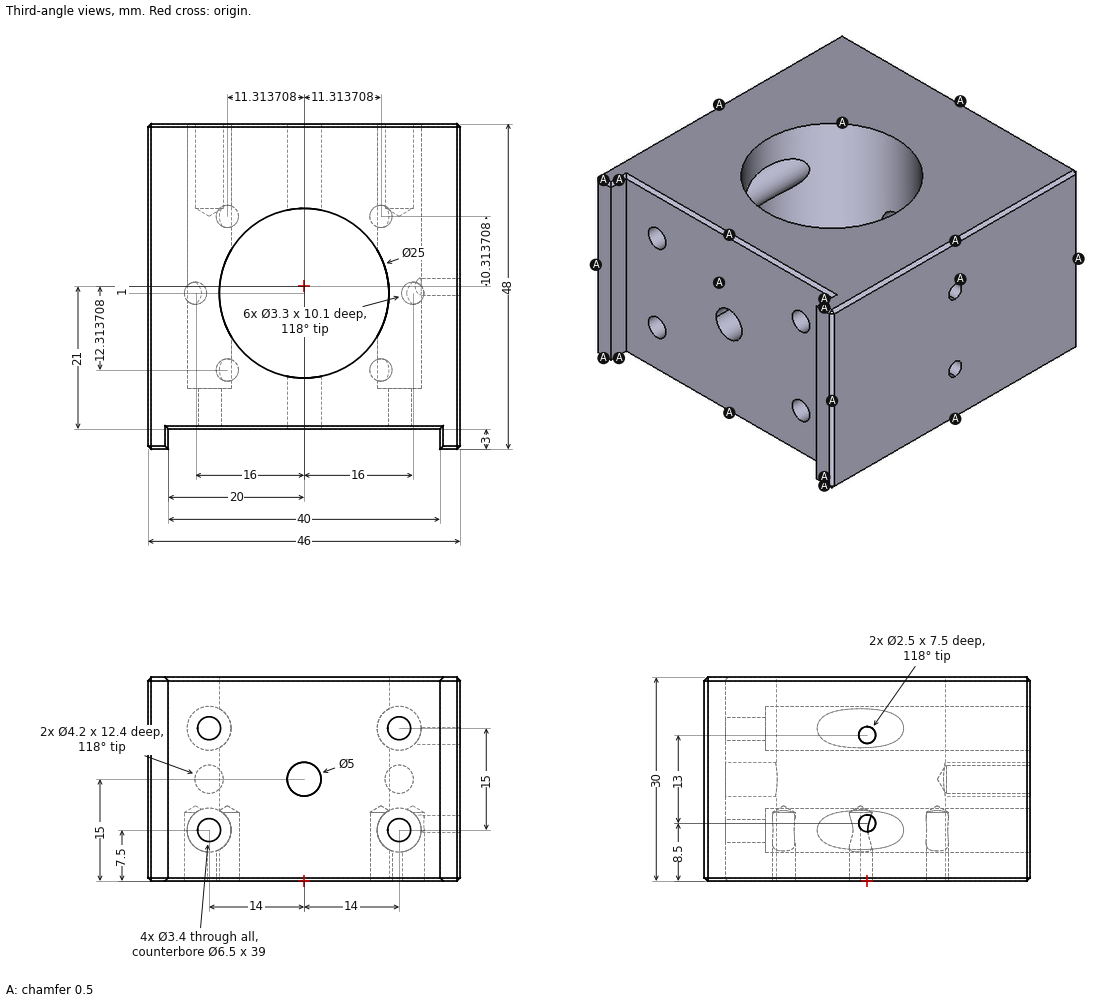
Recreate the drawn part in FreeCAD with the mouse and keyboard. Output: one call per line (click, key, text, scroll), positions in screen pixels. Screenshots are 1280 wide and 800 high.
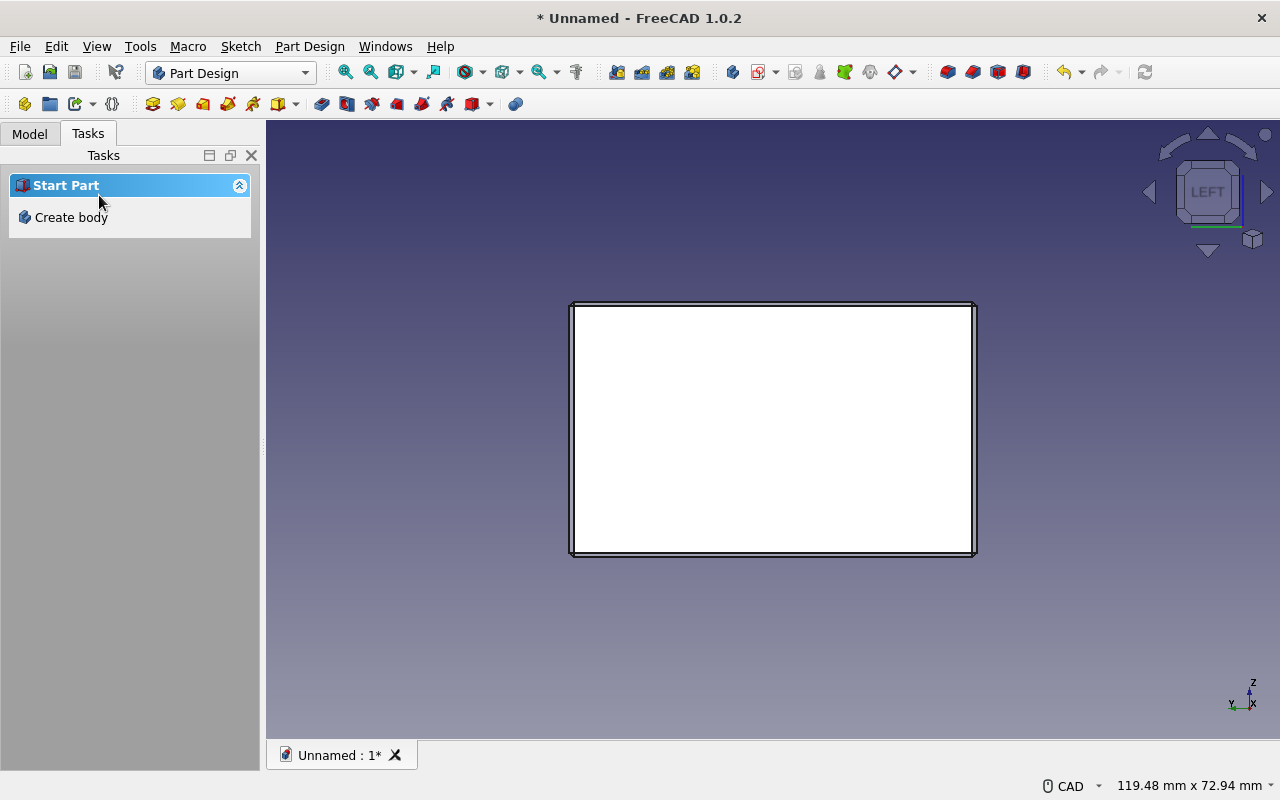
click(346, 72)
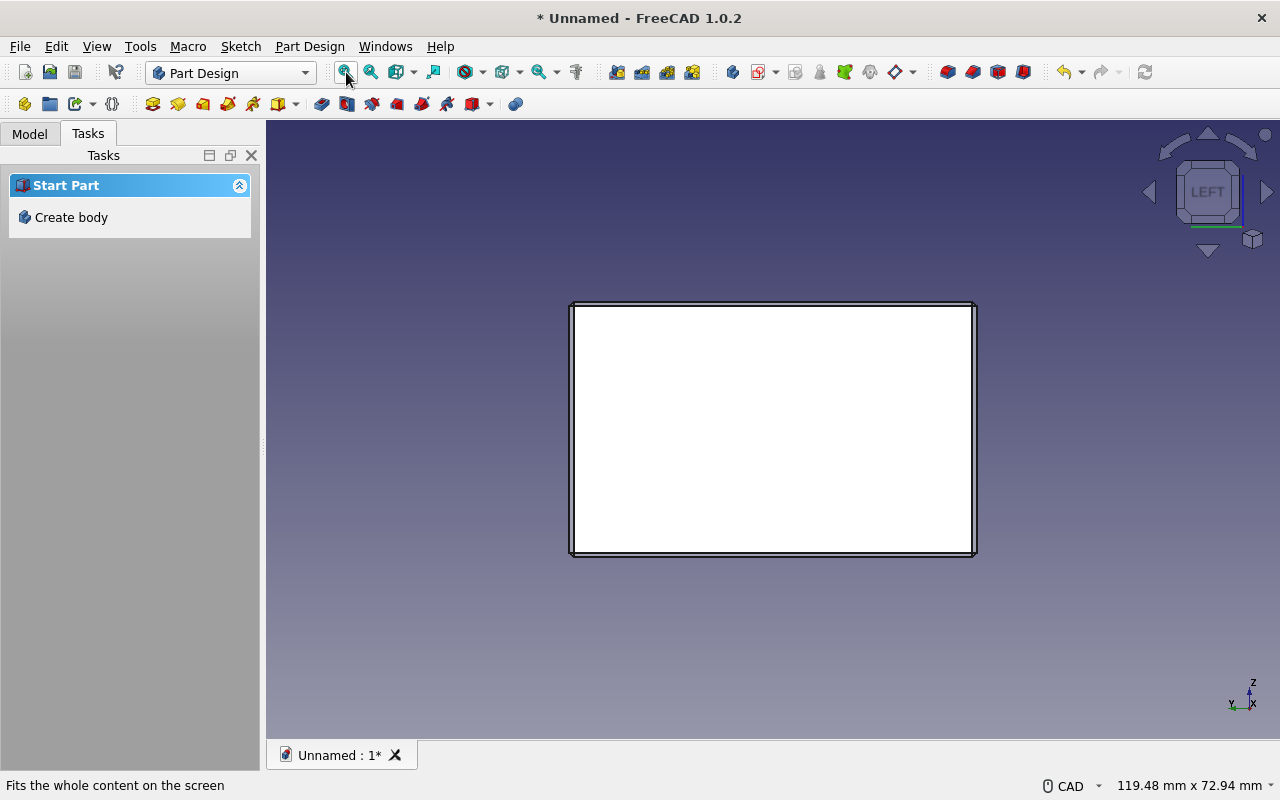
key(4)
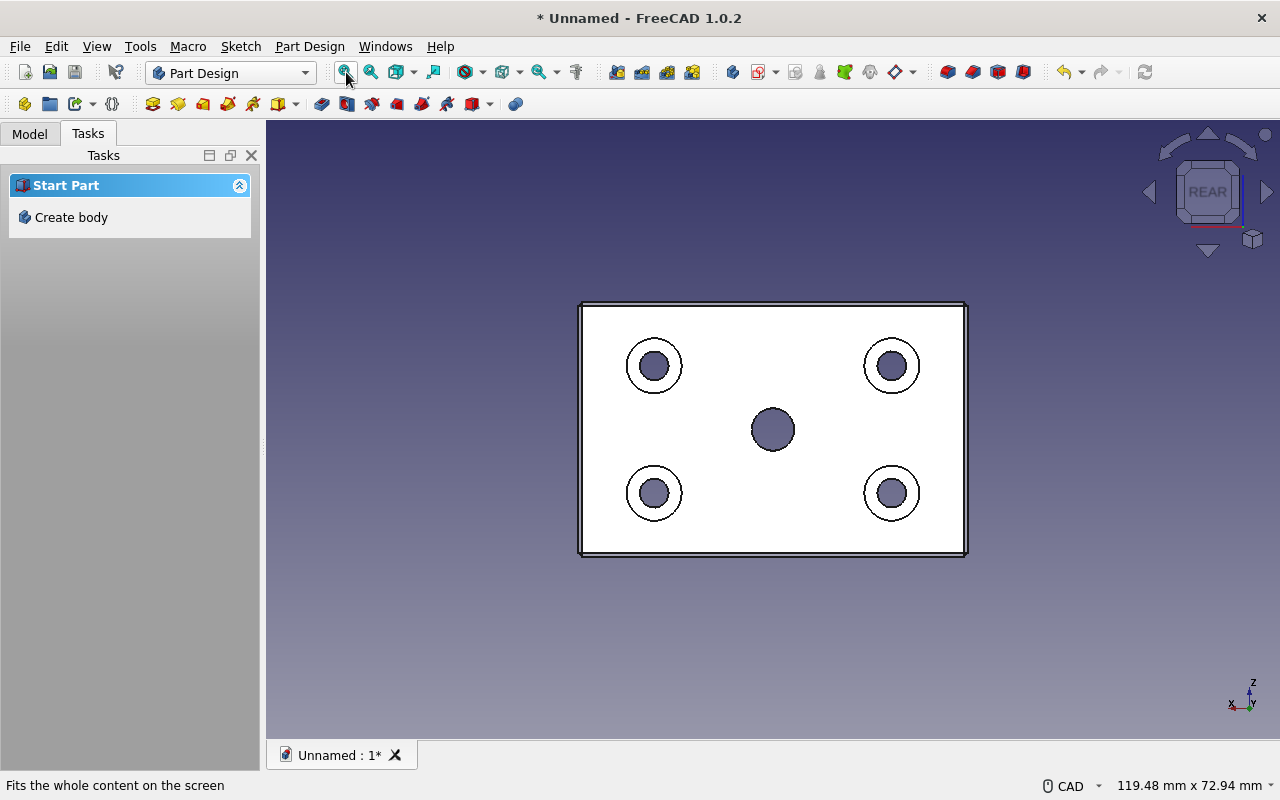
click(346, 72)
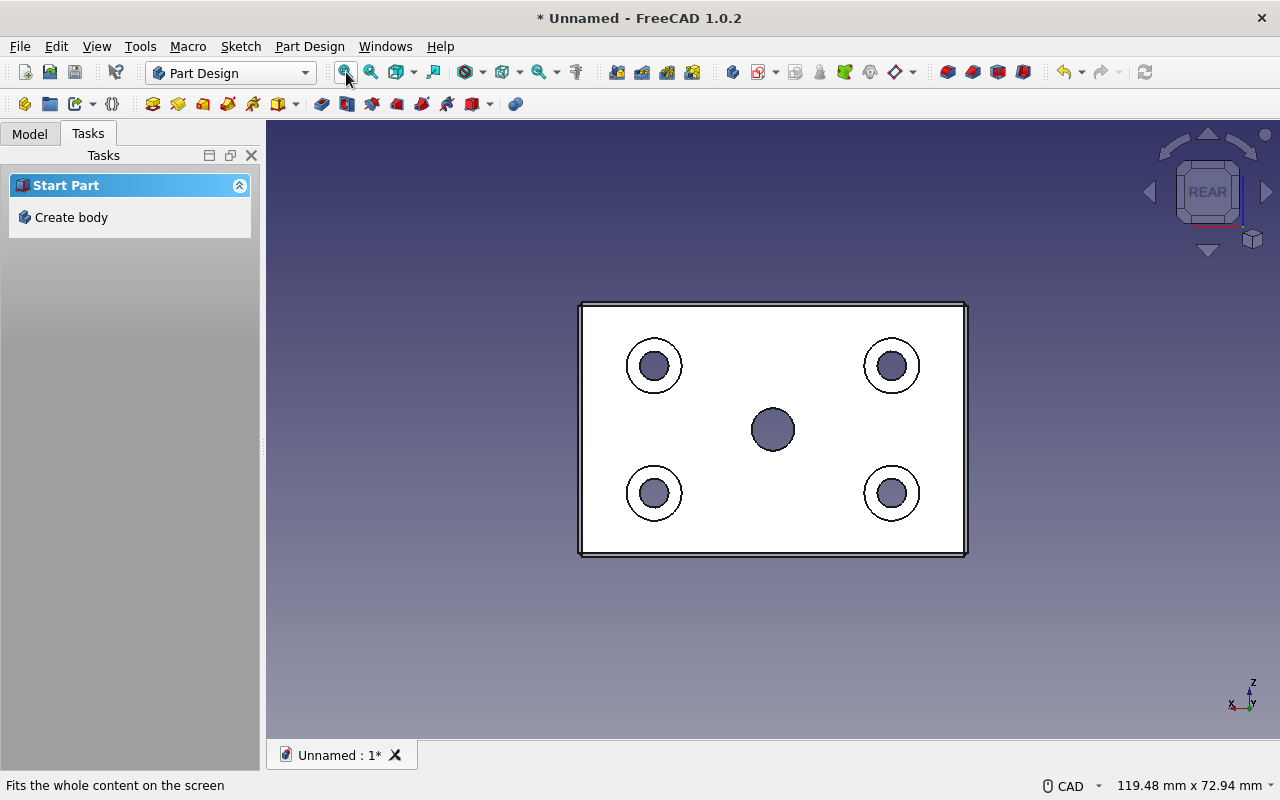
click(773, 358)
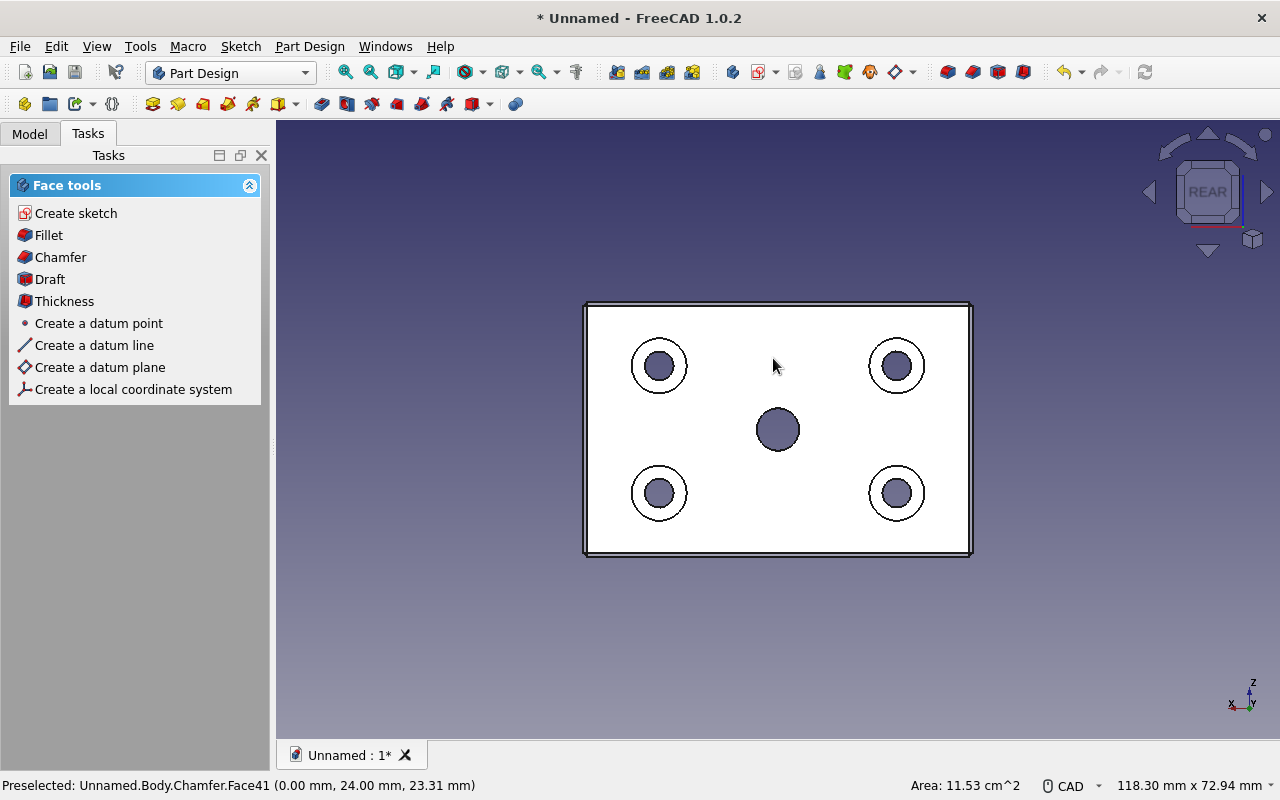
click(758, 72)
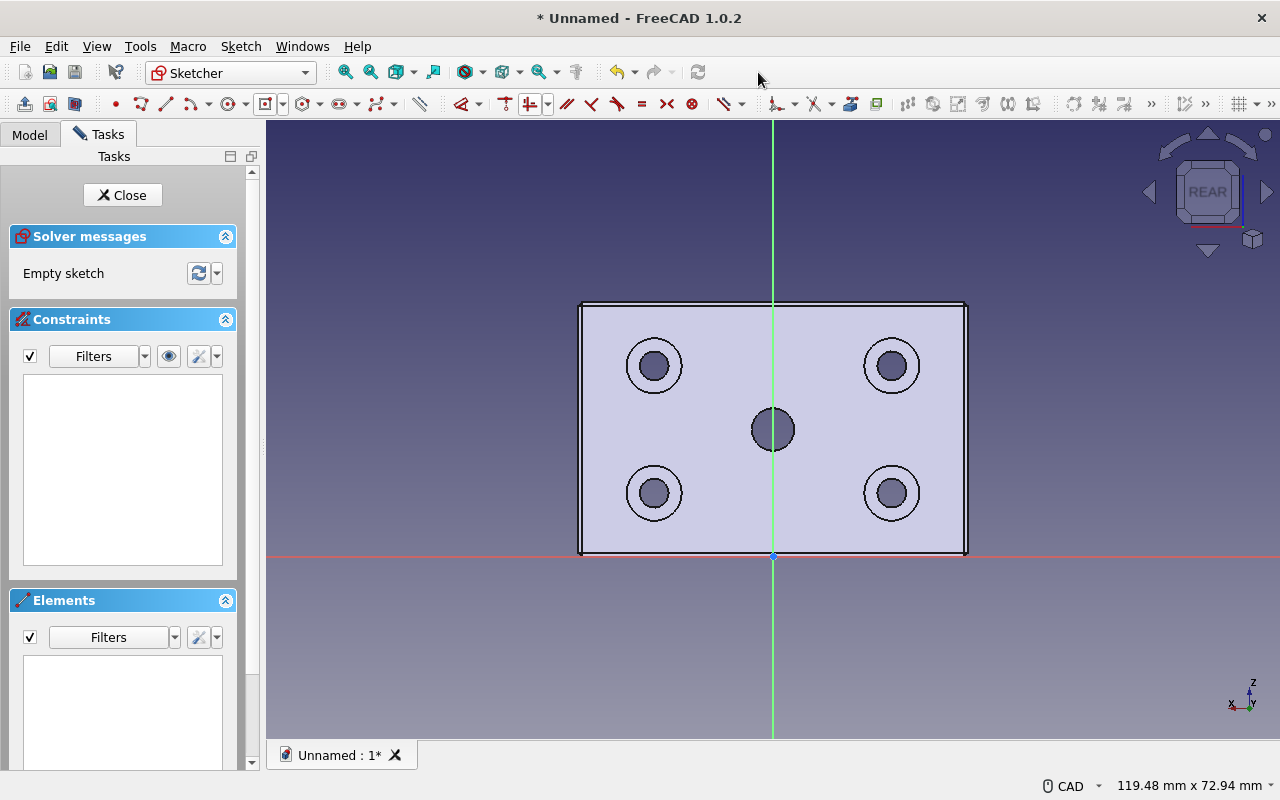
scroll(829, 529, up, 4)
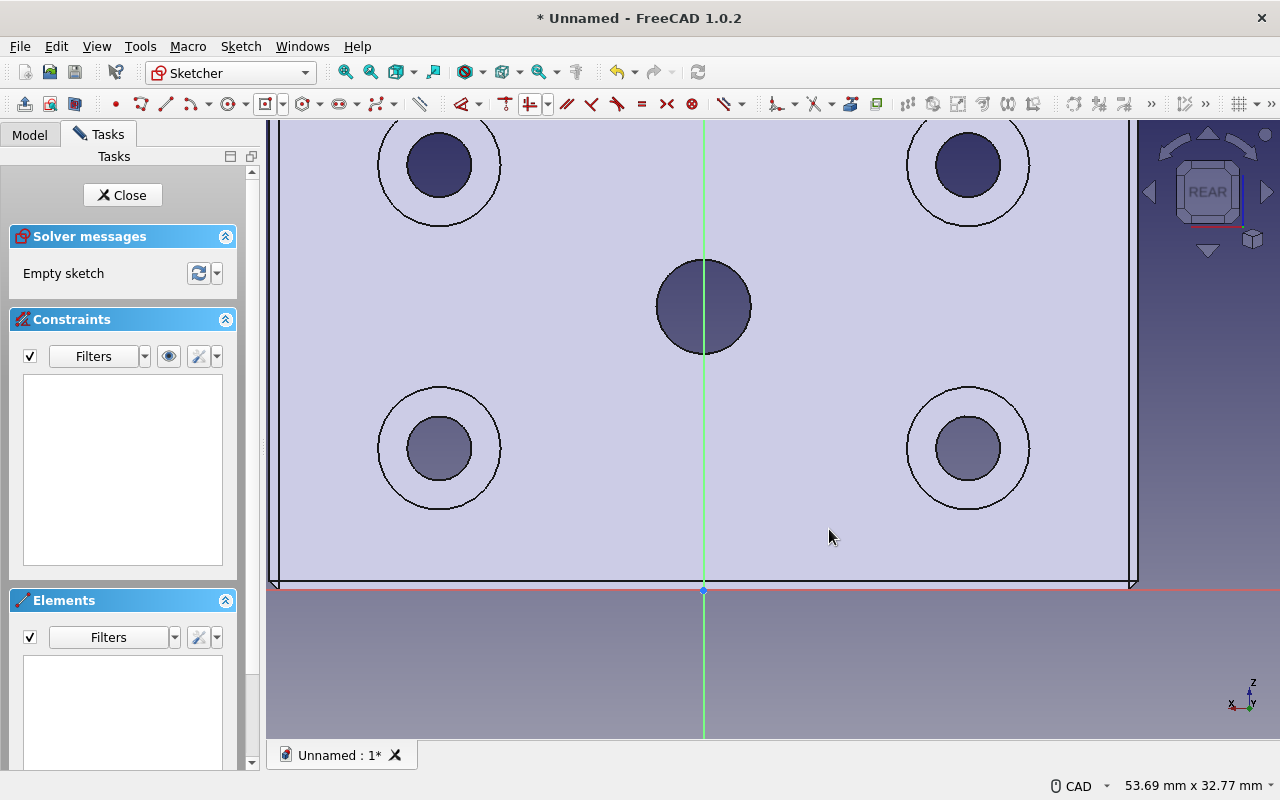
click(228, 104)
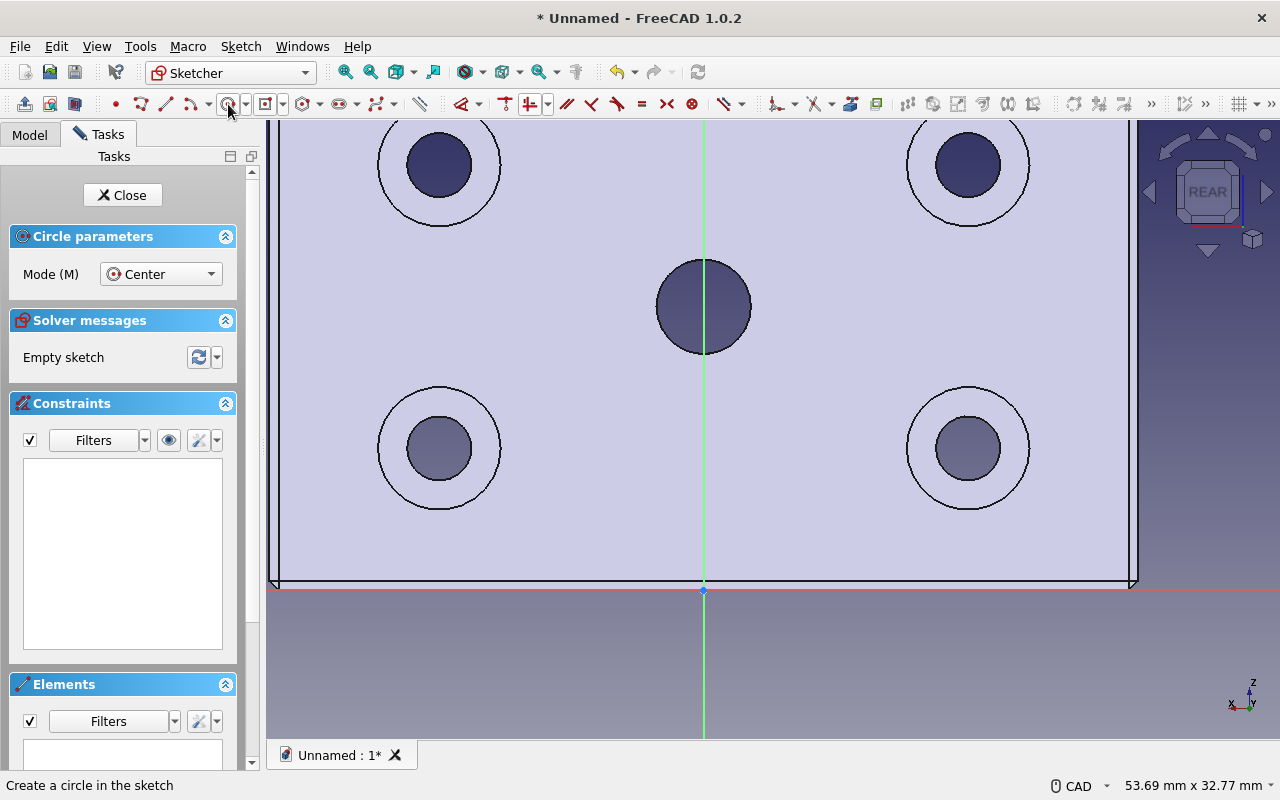
click(968, 307)
move(996, 279)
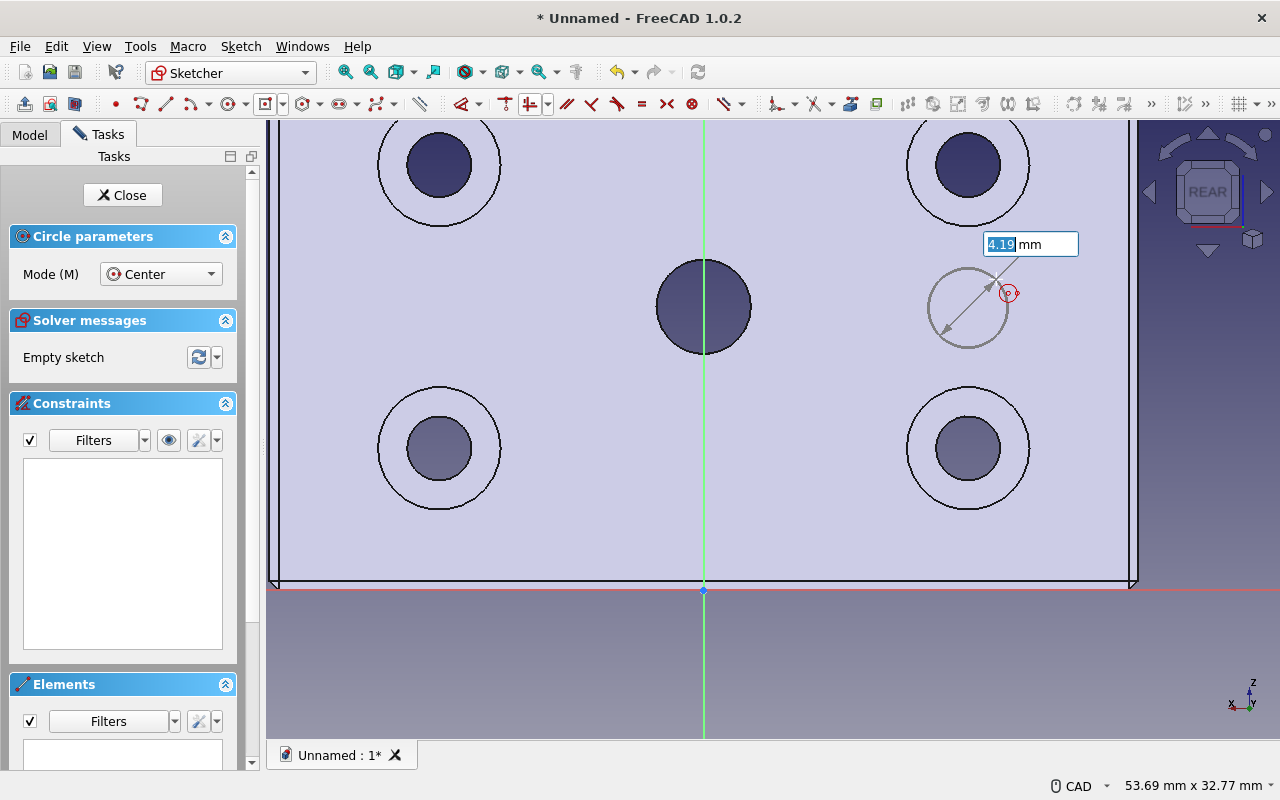
text(4.2)
key(Return)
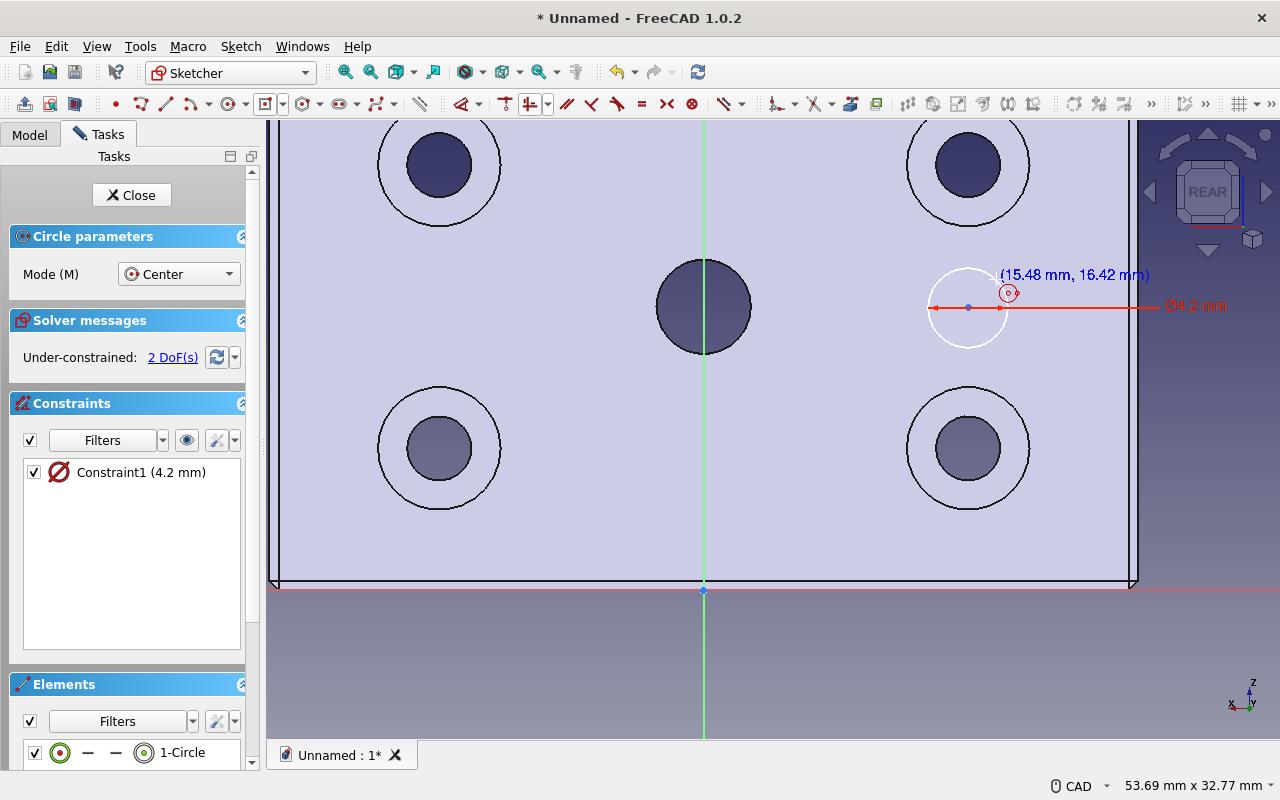
click(439, 307)
move(467, 279)